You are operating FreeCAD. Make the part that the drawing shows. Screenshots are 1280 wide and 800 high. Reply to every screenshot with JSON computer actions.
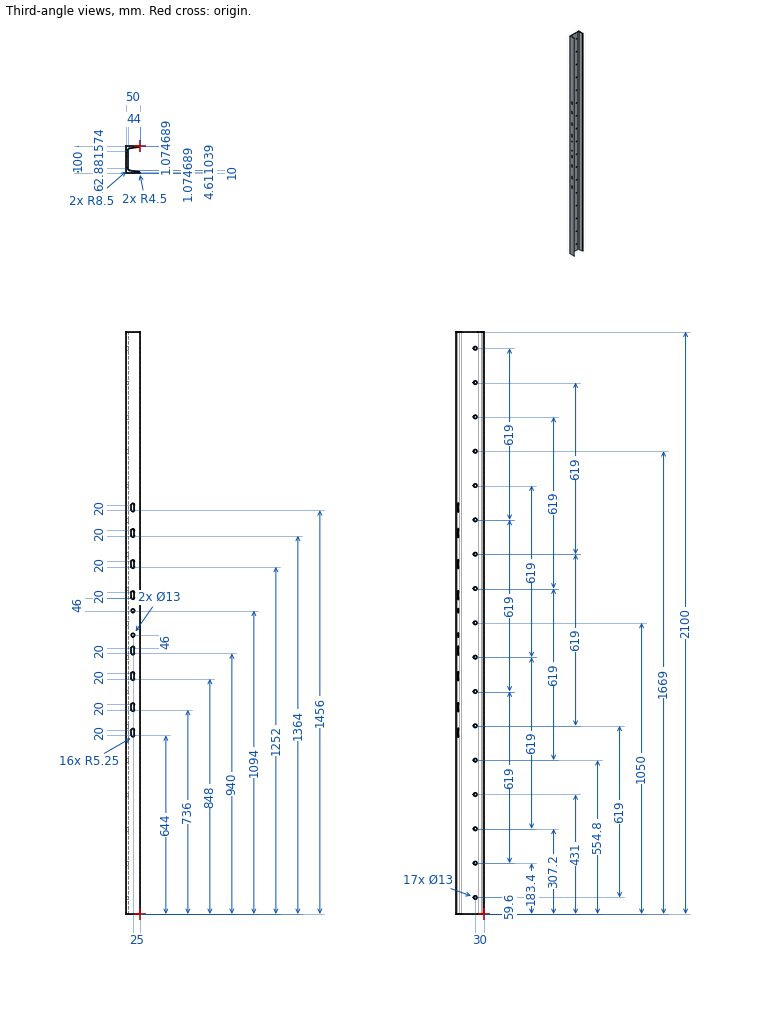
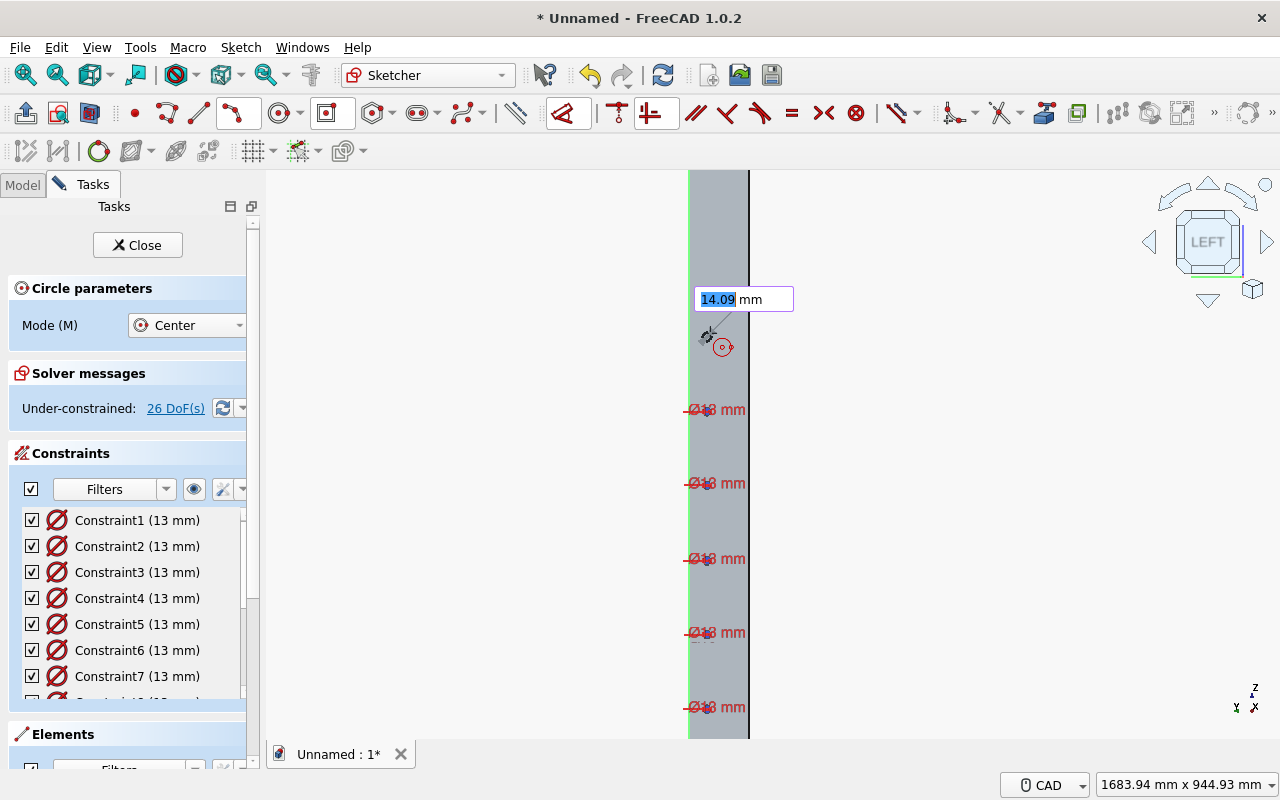
{"action": "type", "text": "13"}
{"action": "key", "text": "Return"}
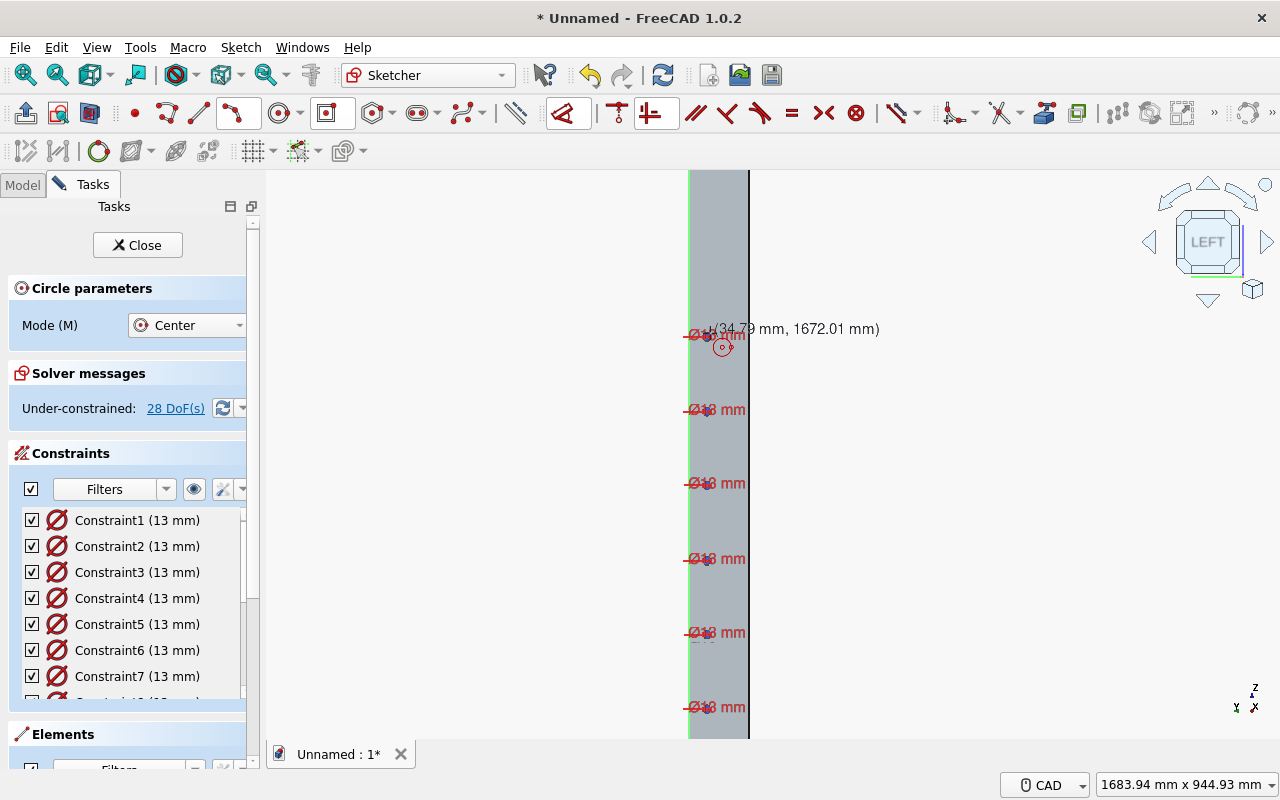
{"action": "scroll", "coordinate": [707, 261], "scroll_direction": "up", "scroll_amount": 9}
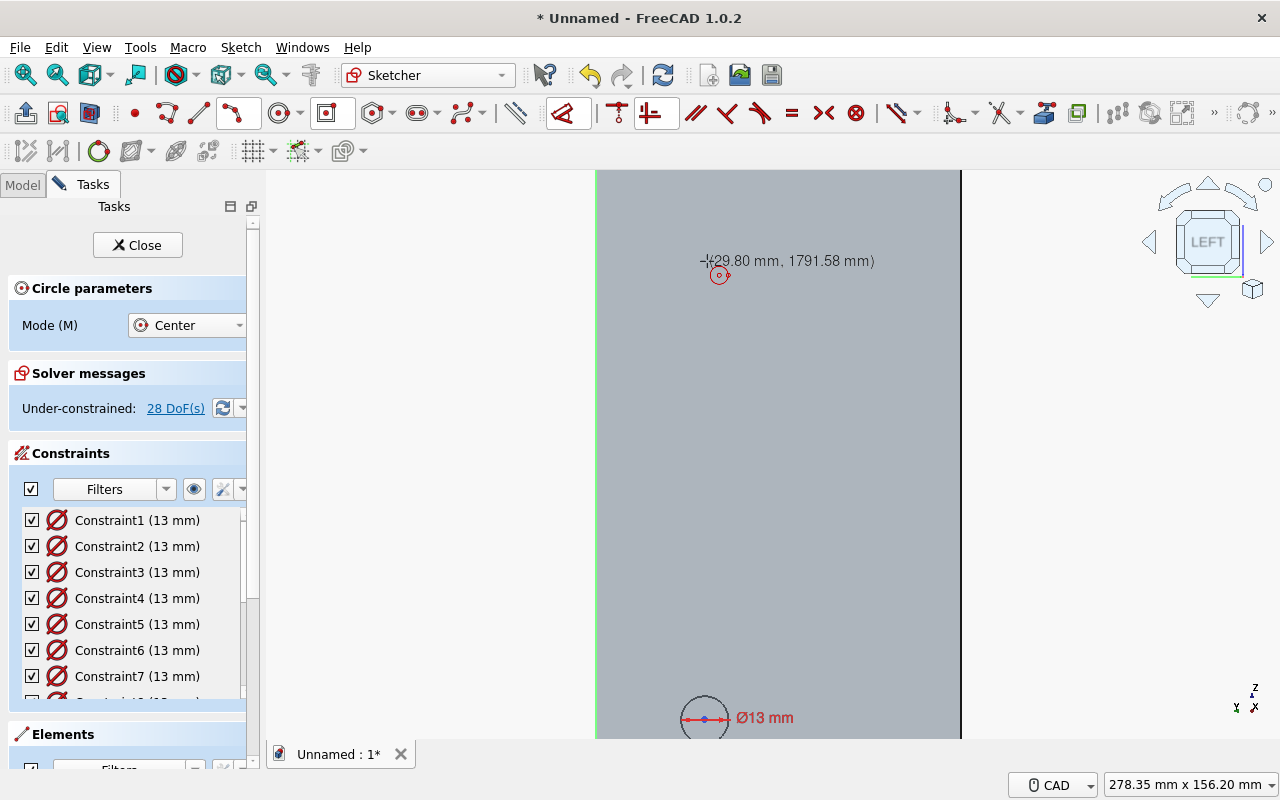
{"action": "scroll", "coordinate": [707, 318], "scroll_direction": "down", "scroll_amount": 15}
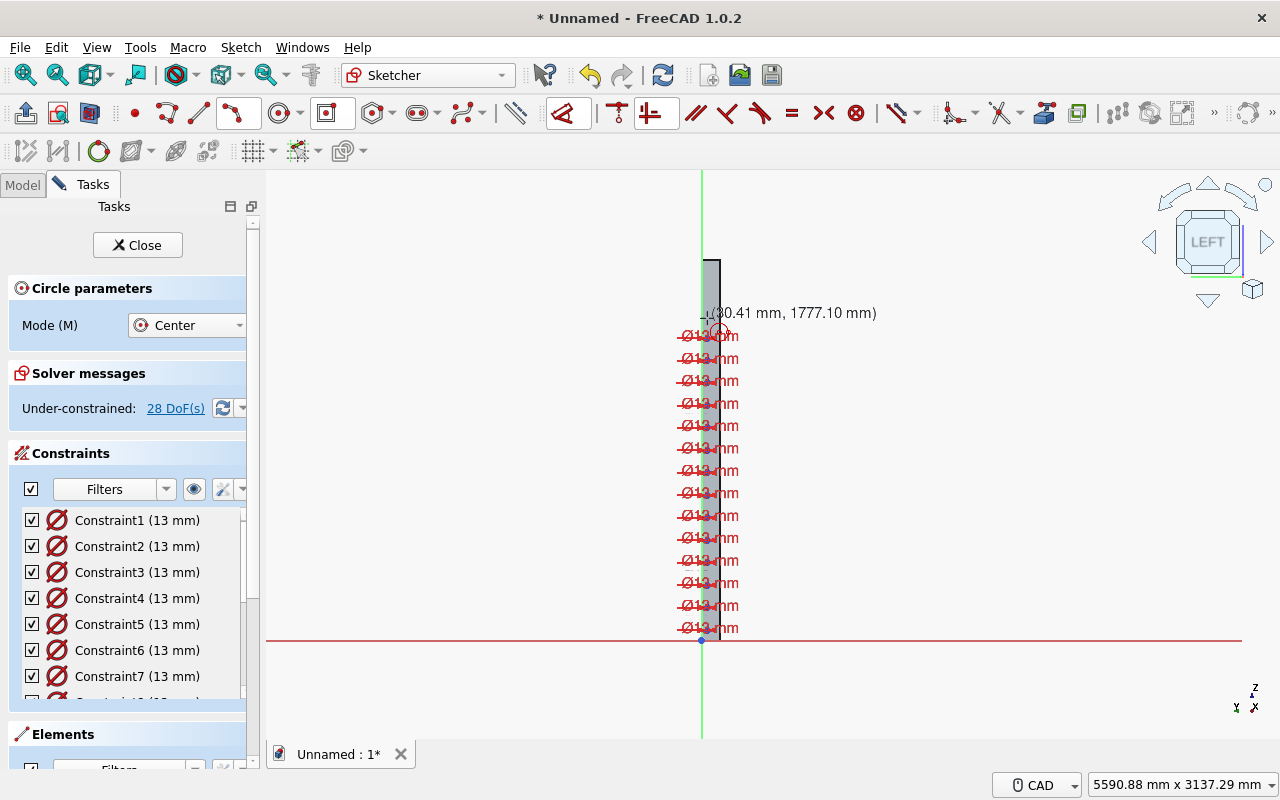
{"action": "scroll", "coordinate": [707, 315], "scroll_direction": "up", "scroll_amount": 6}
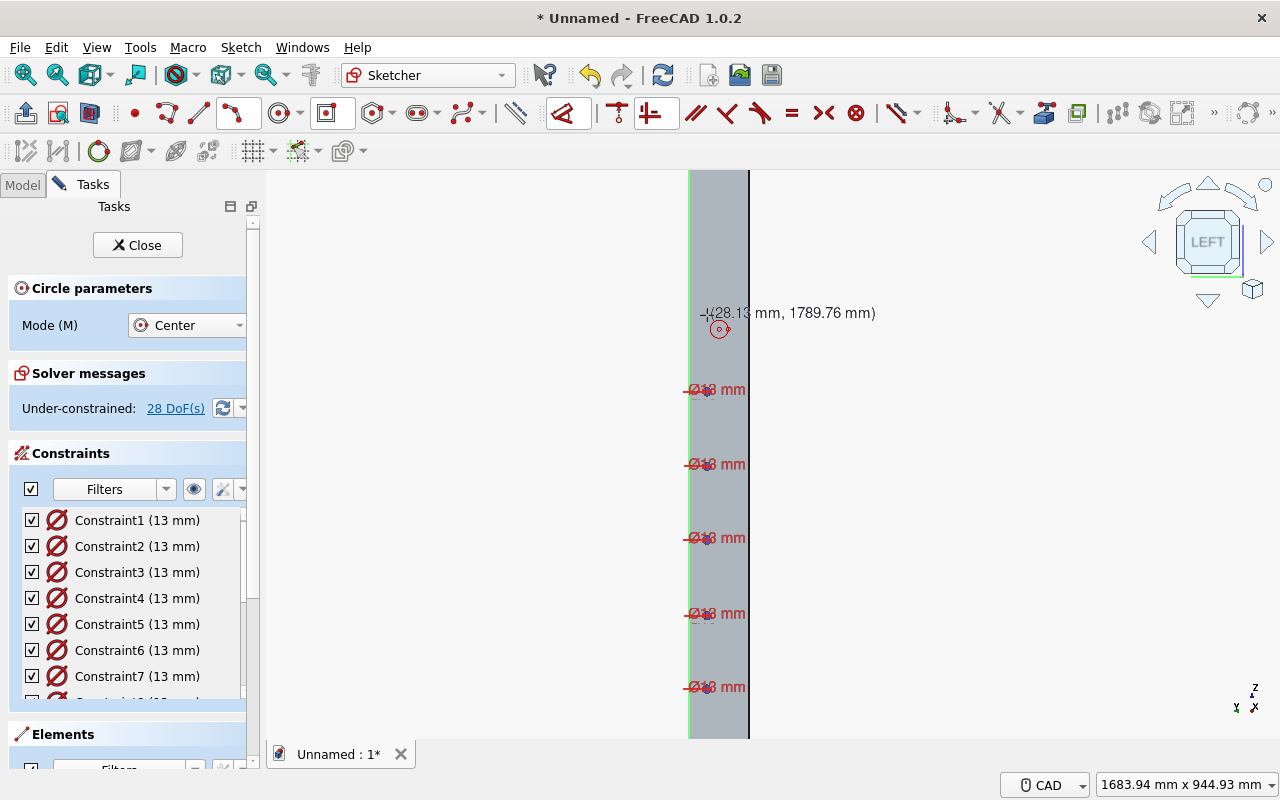
{"action": "left_click", "coordinate": [707, 316]}
{"action": "mouse_move", "coordinate": [710, 313]}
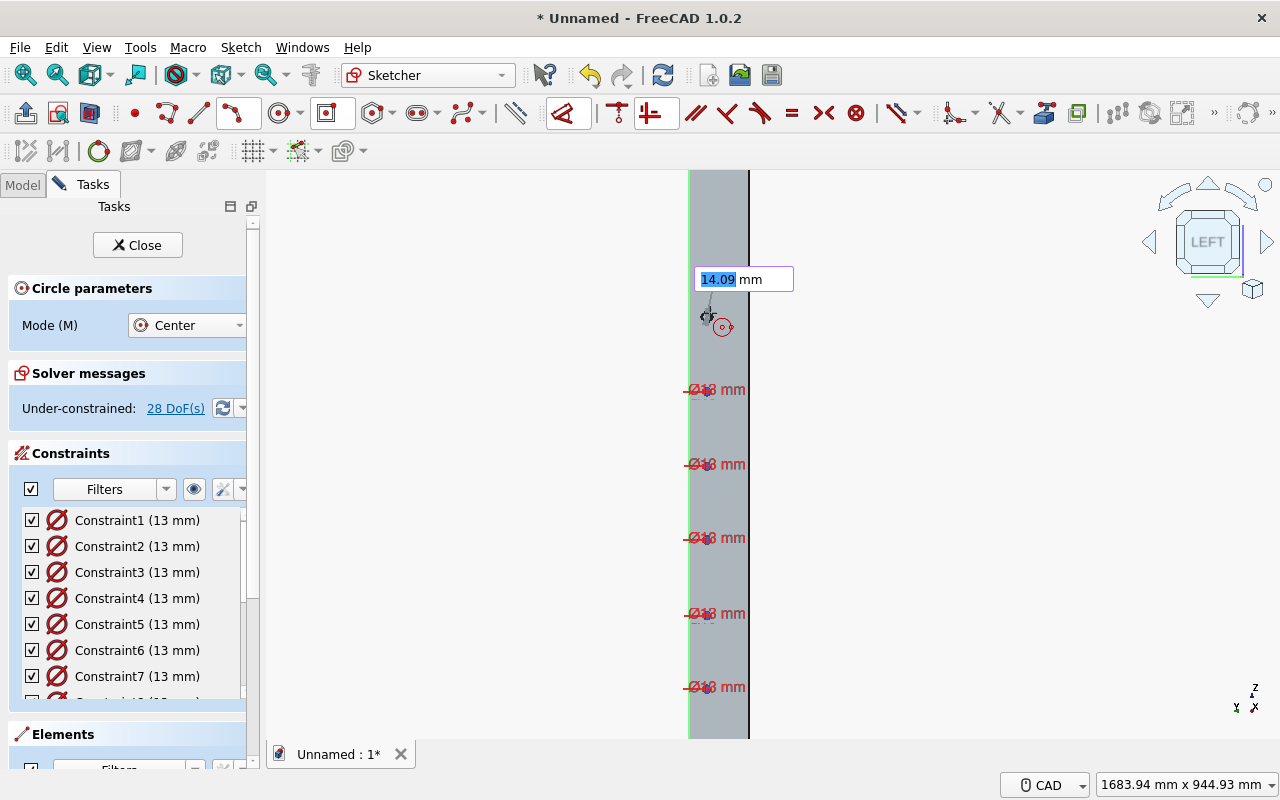
{"action": "type", "text": "13"}
{"action": "key", "text": "Return"}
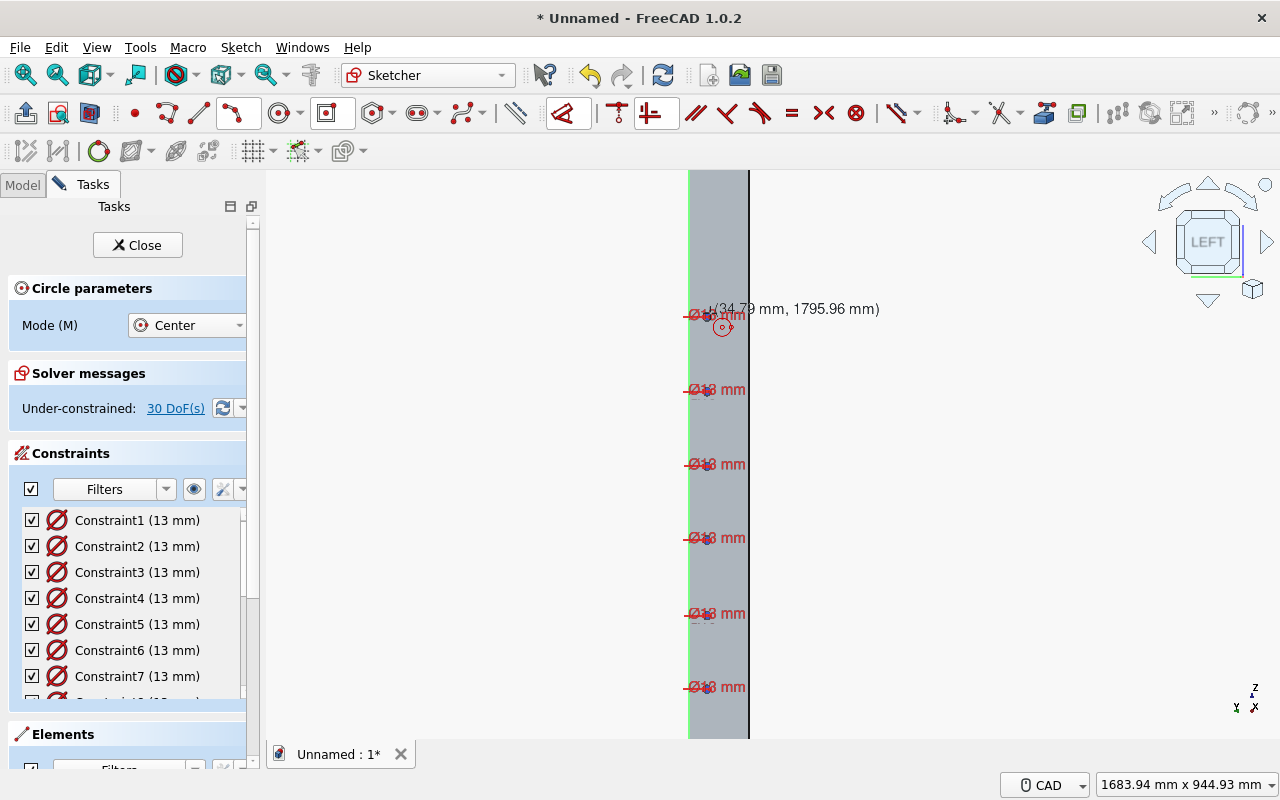
{"action": "scroll", "coordinate": [707, 241], "scroll_direction": "up", "scroll_amount": 9}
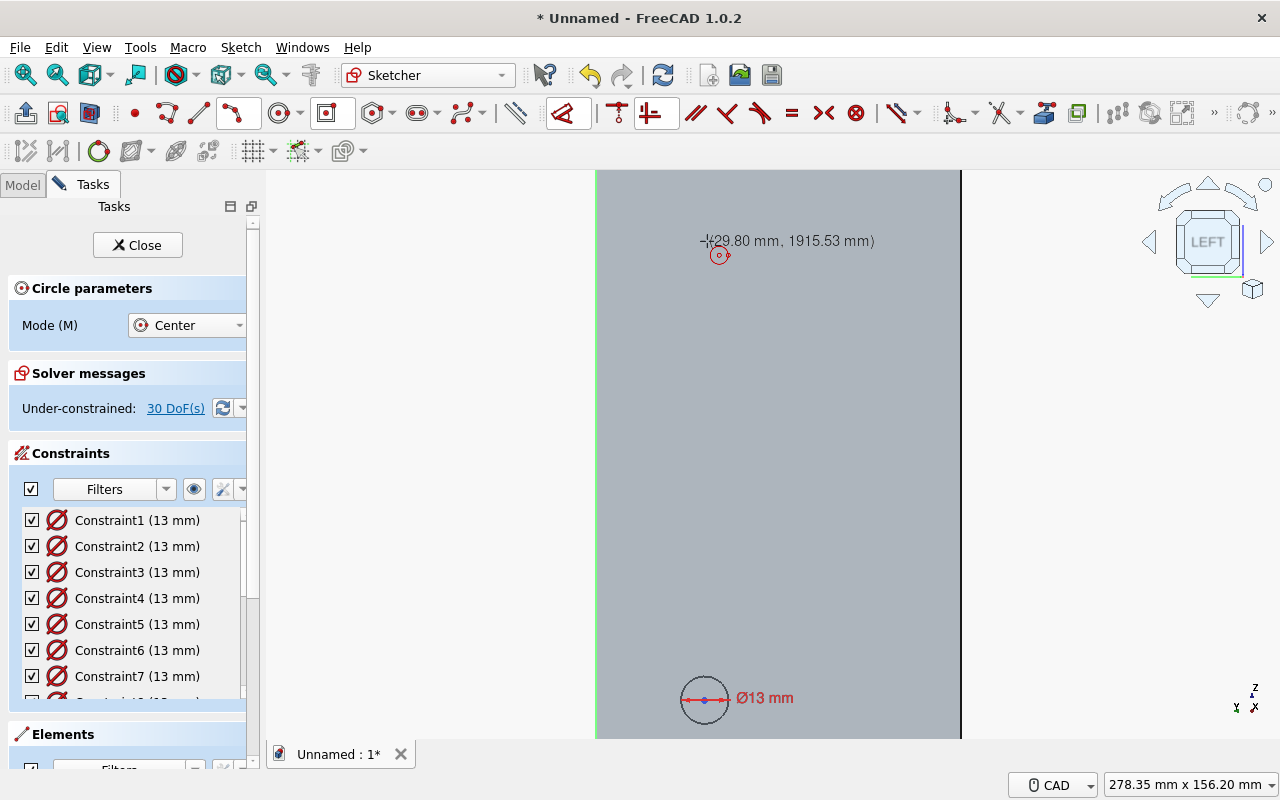
{"action": "scroll", "coordinate": [707, 295], "scroll_direction": "down", "scroll_amount": 15}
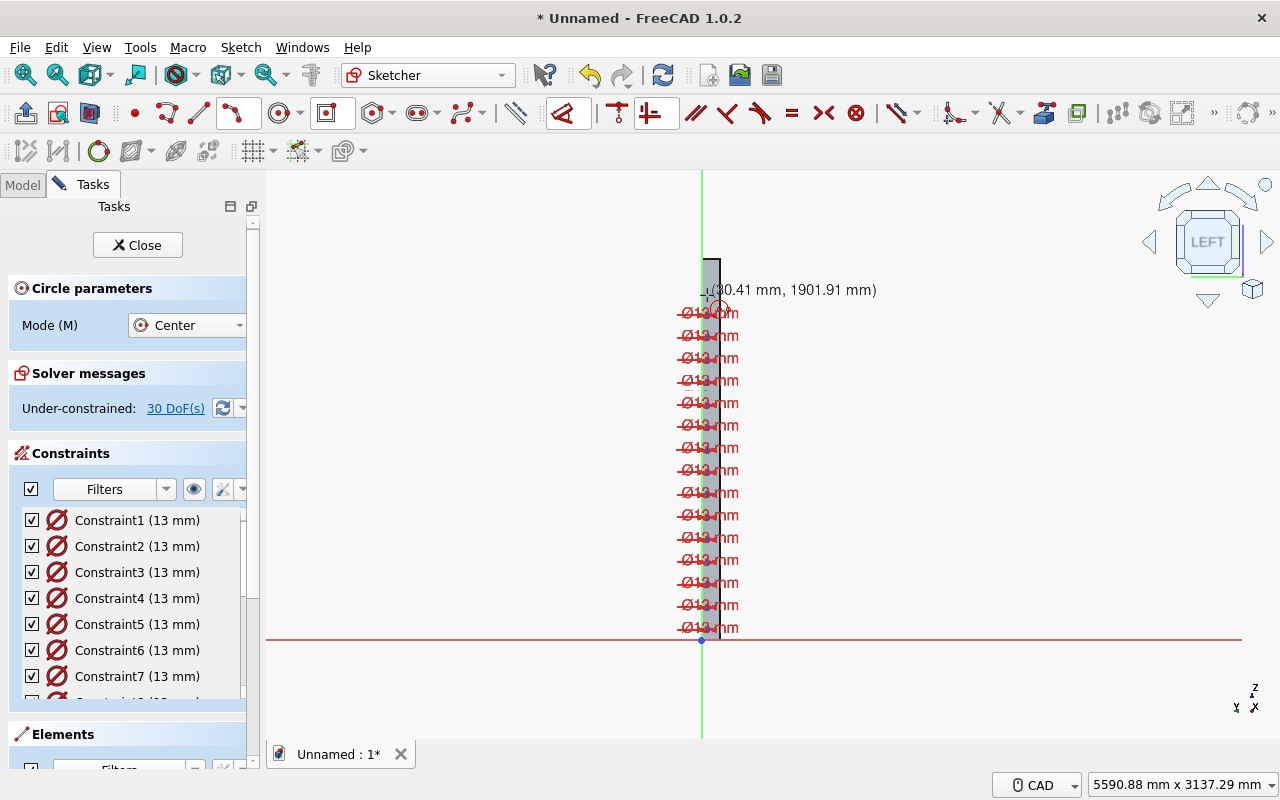
{"action": "scroll", "coordinate": [707, 293], "scroll_direction": "up", "scroll_amount": 6}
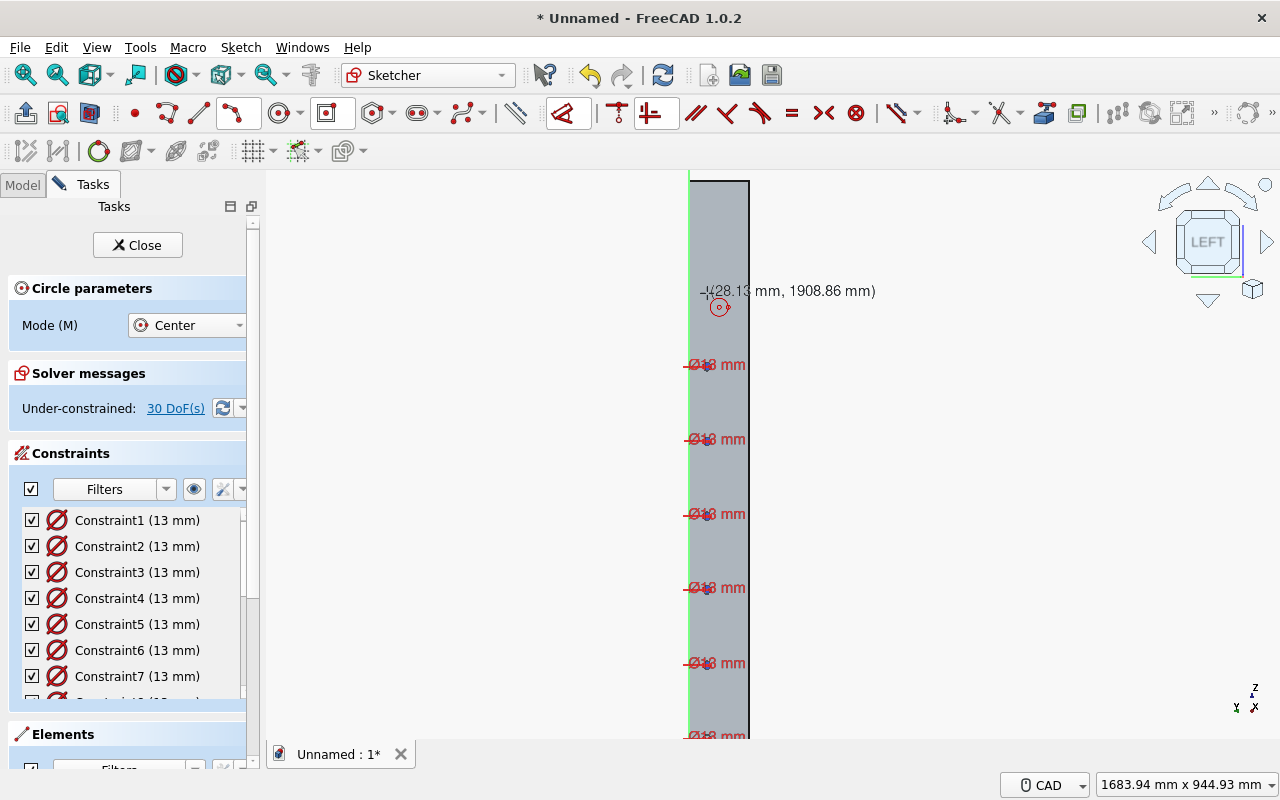
{"action": "left_click", "coordinate": [707, 291]}
{"action": "mouse_move", "coordinate": [710, 288]}